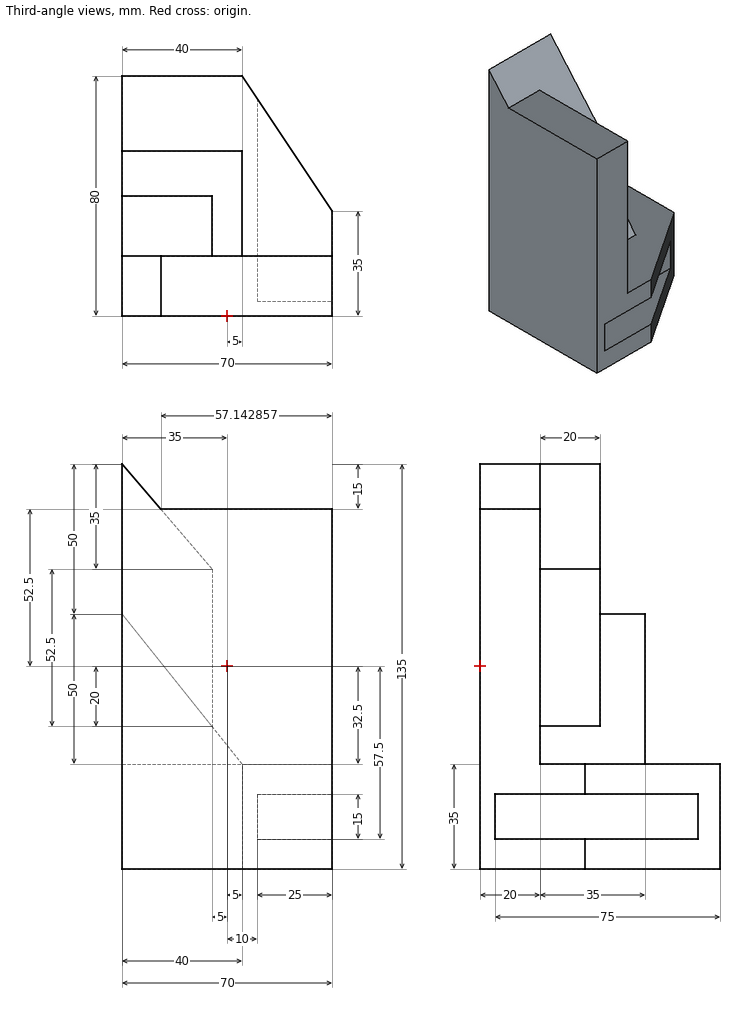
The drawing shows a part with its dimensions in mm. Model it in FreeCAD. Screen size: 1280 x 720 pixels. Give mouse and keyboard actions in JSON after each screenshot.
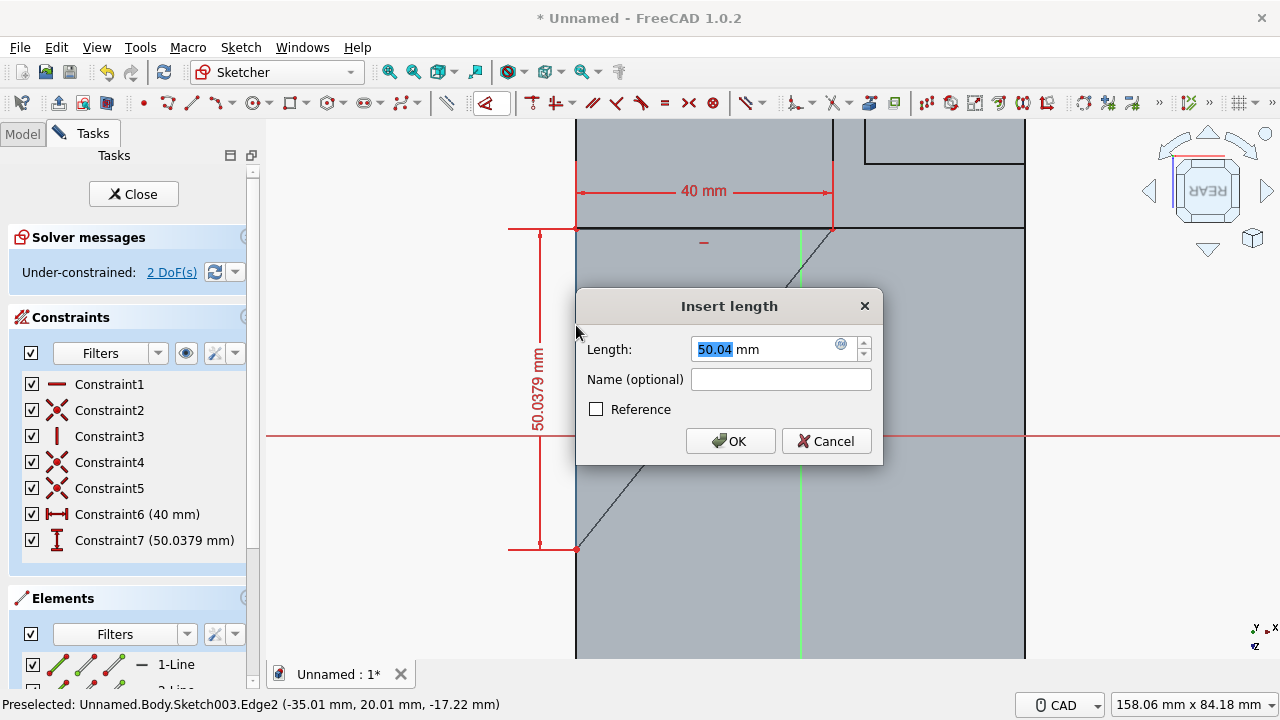
{"action": "type", "text": "50"}
{"action": "key", "text": "Return"}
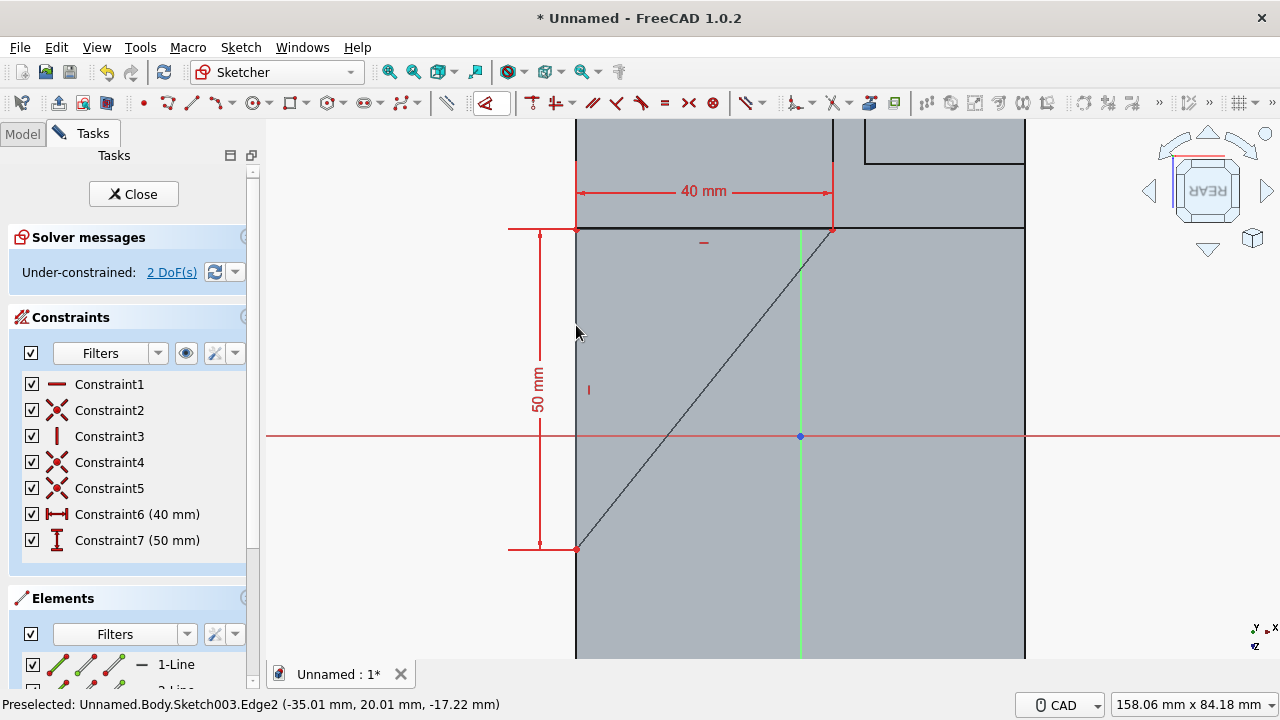
{"action": "scroll", "coordinate": [833, 229], "scroll_direction": "up", "scroll_amount": 2}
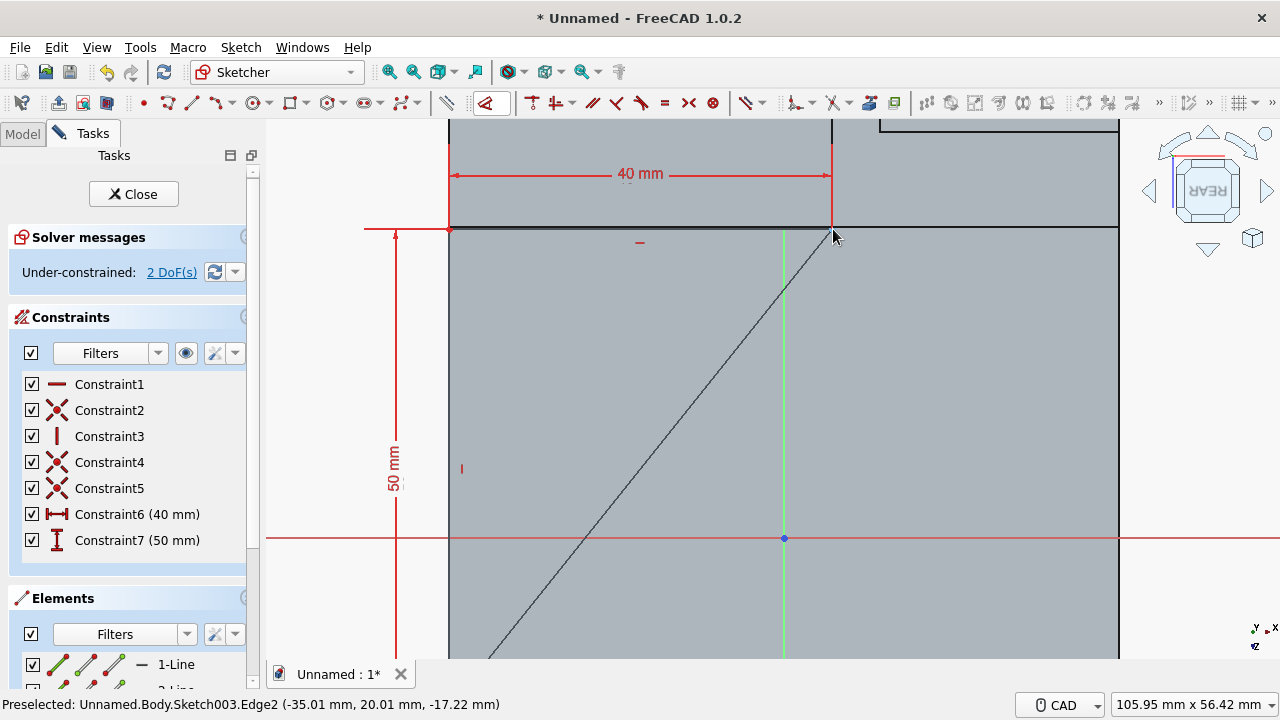
{"action": "left_click", "coordinate": [832, 229]}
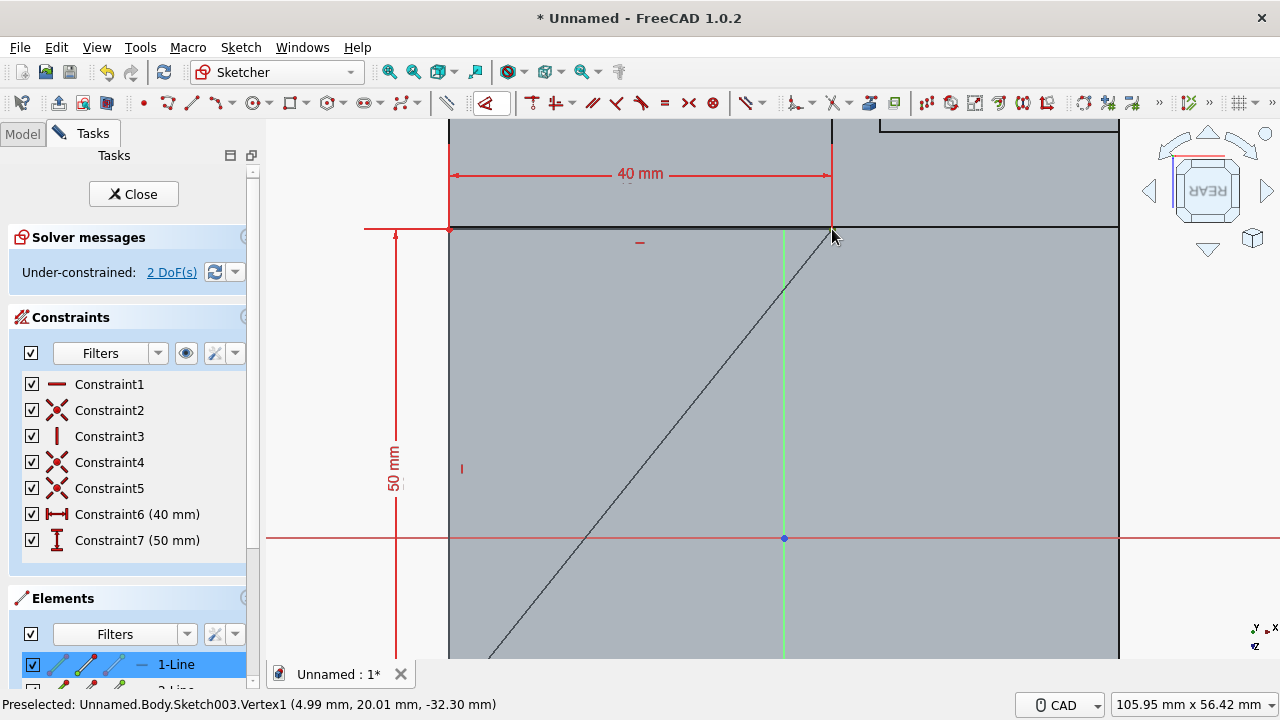
{"action": "left_click", "coordinate": [504, 104]}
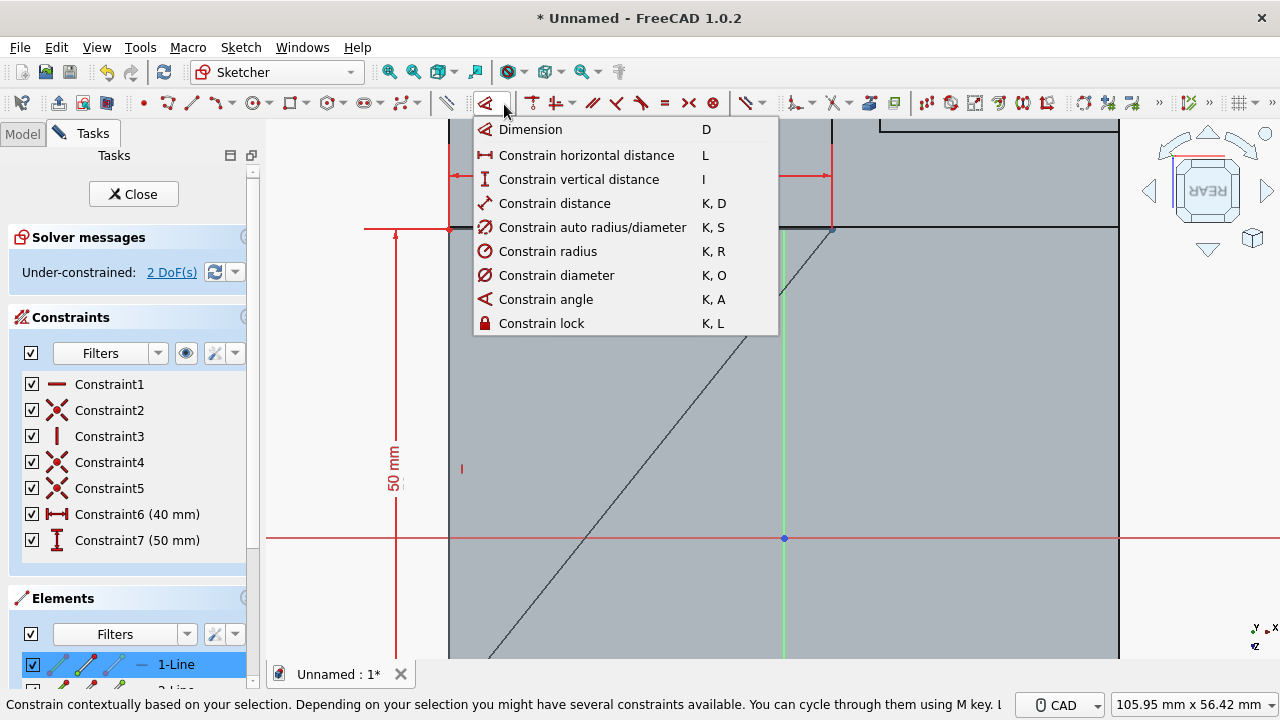
{"action": "left_click", "coordinate": [626, 155]}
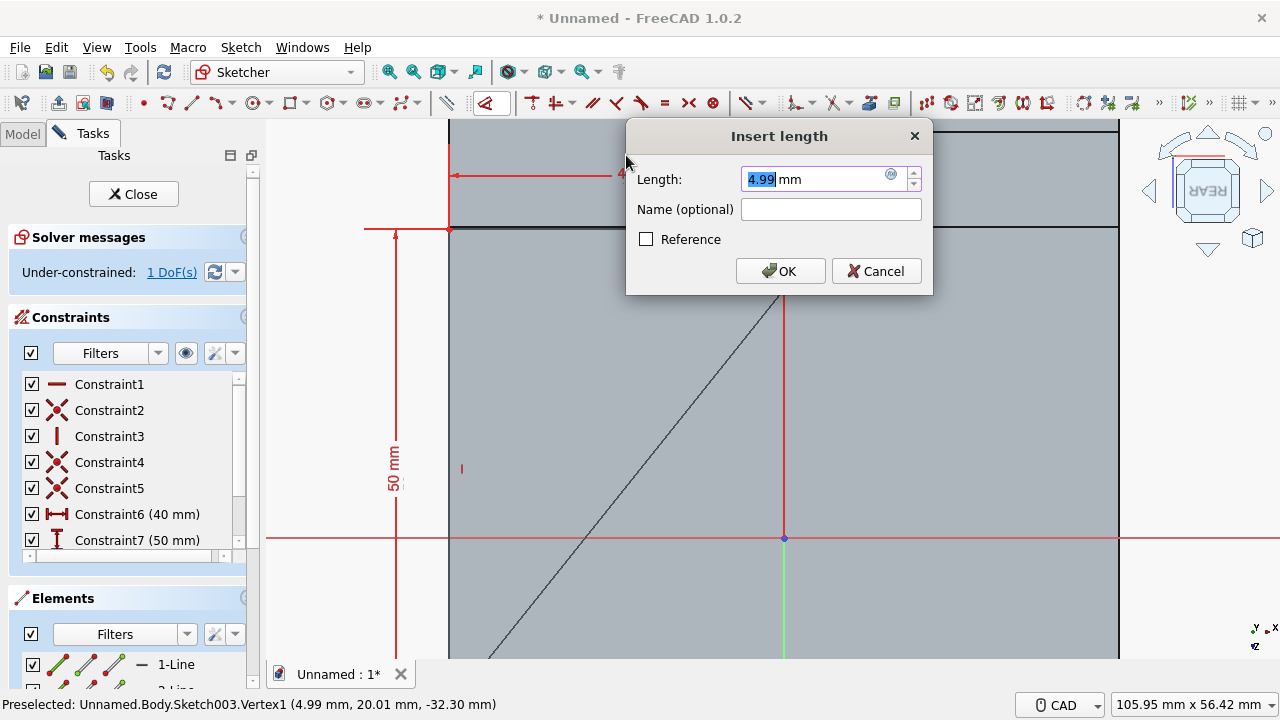
{"action": "type", "text": "5"}
{"action": "key", "text": "Return"}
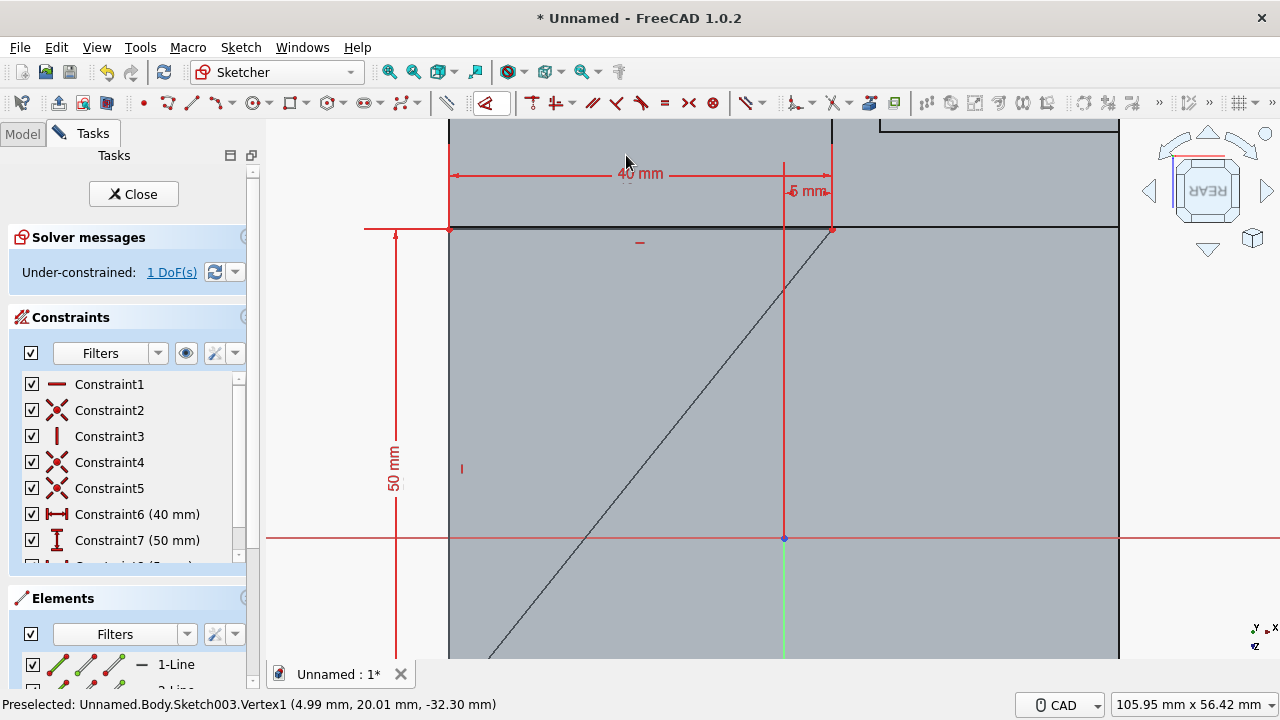
{"action": "left_click", "coordinate": [832, 229]}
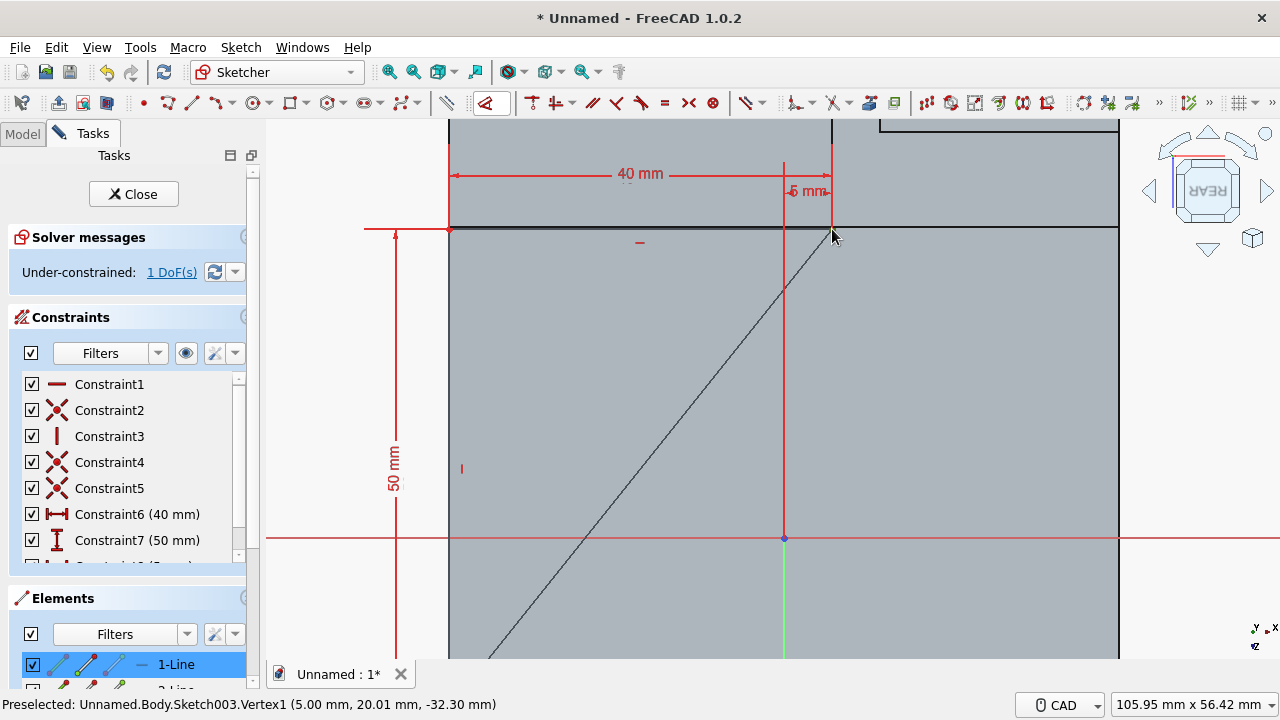
{"action": "left_click", "coordinate": [504, 104]}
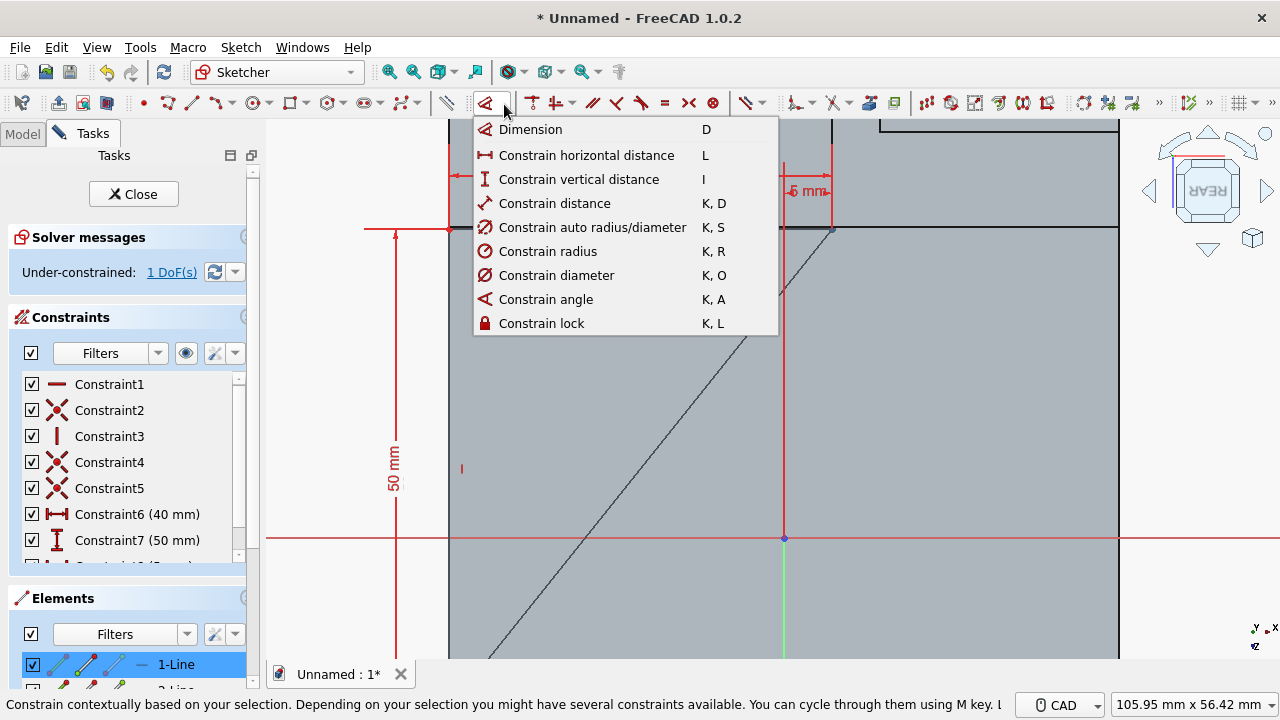
{"action": "left_click", "coordinate": [626, 179]}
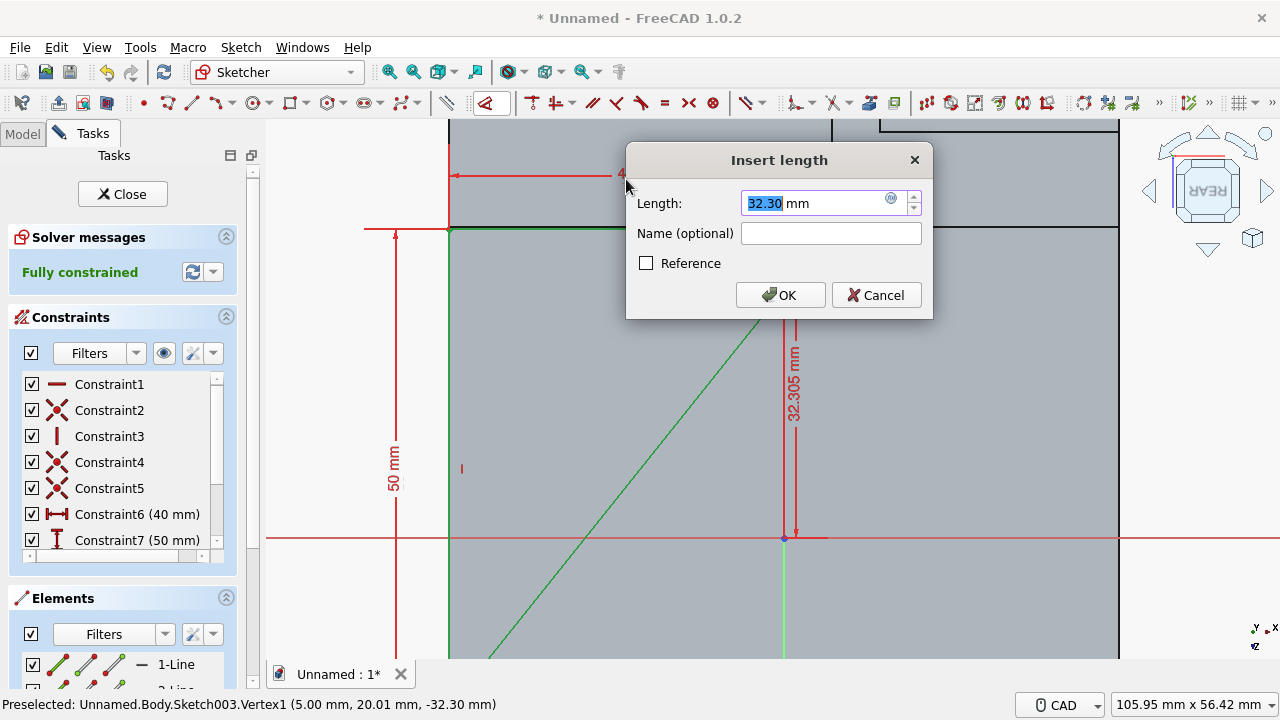
{"action": "type", "text": "32.5"}
{"action": "key", "text": "Return"}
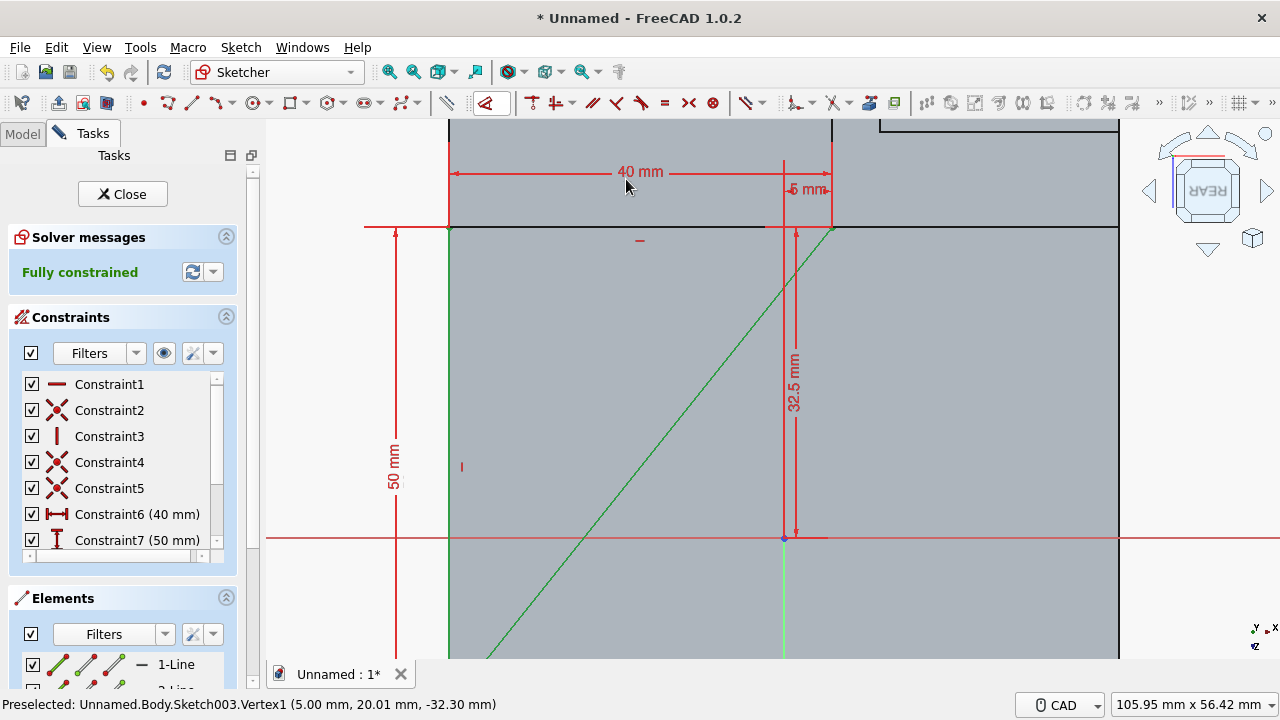
{"action": "left_click", "coordinate": [123, 194]}